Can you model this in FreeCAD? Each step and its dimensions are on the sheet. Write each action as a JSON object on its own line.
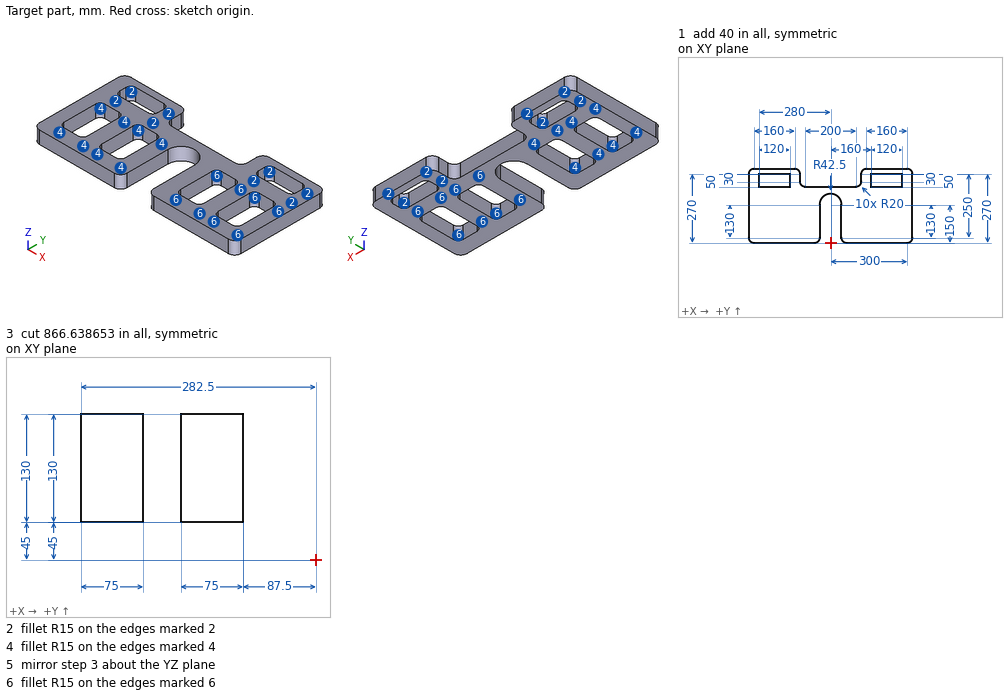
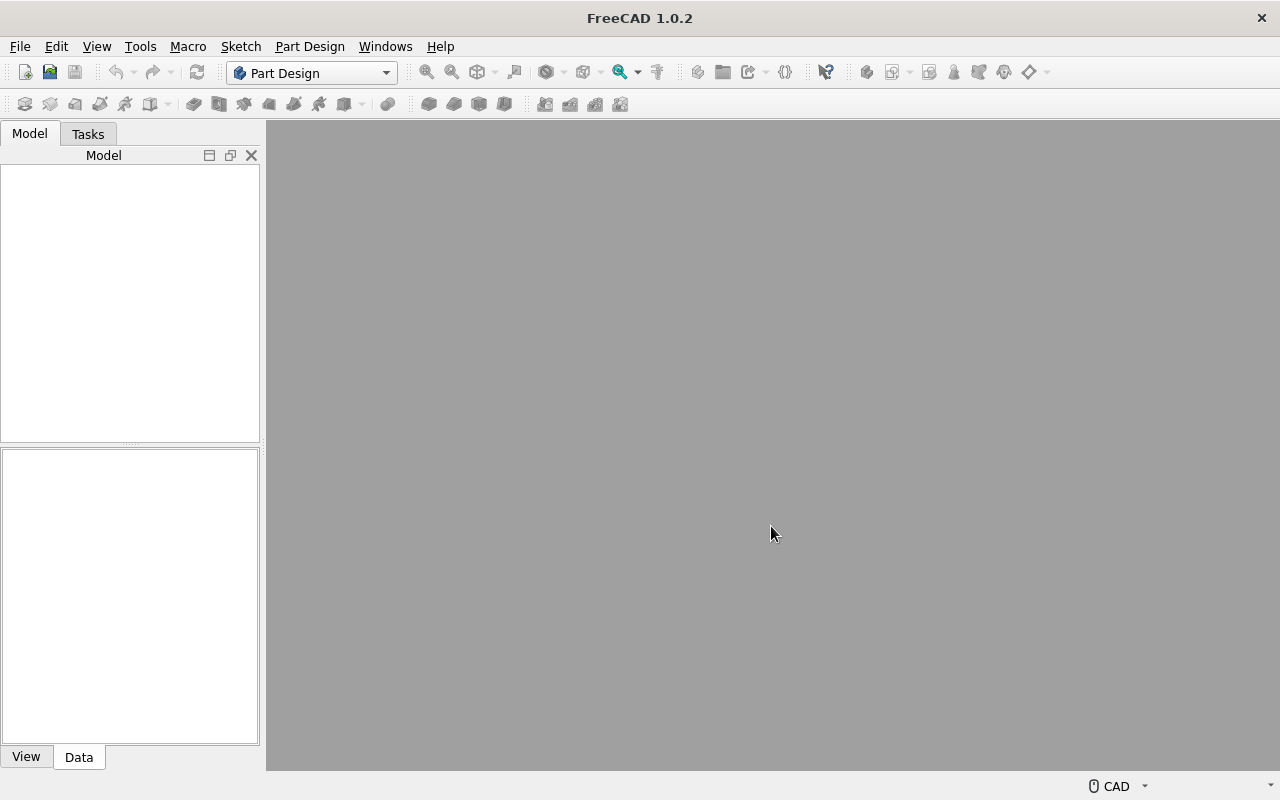
{"action": "key", "text": "ctrl+n"}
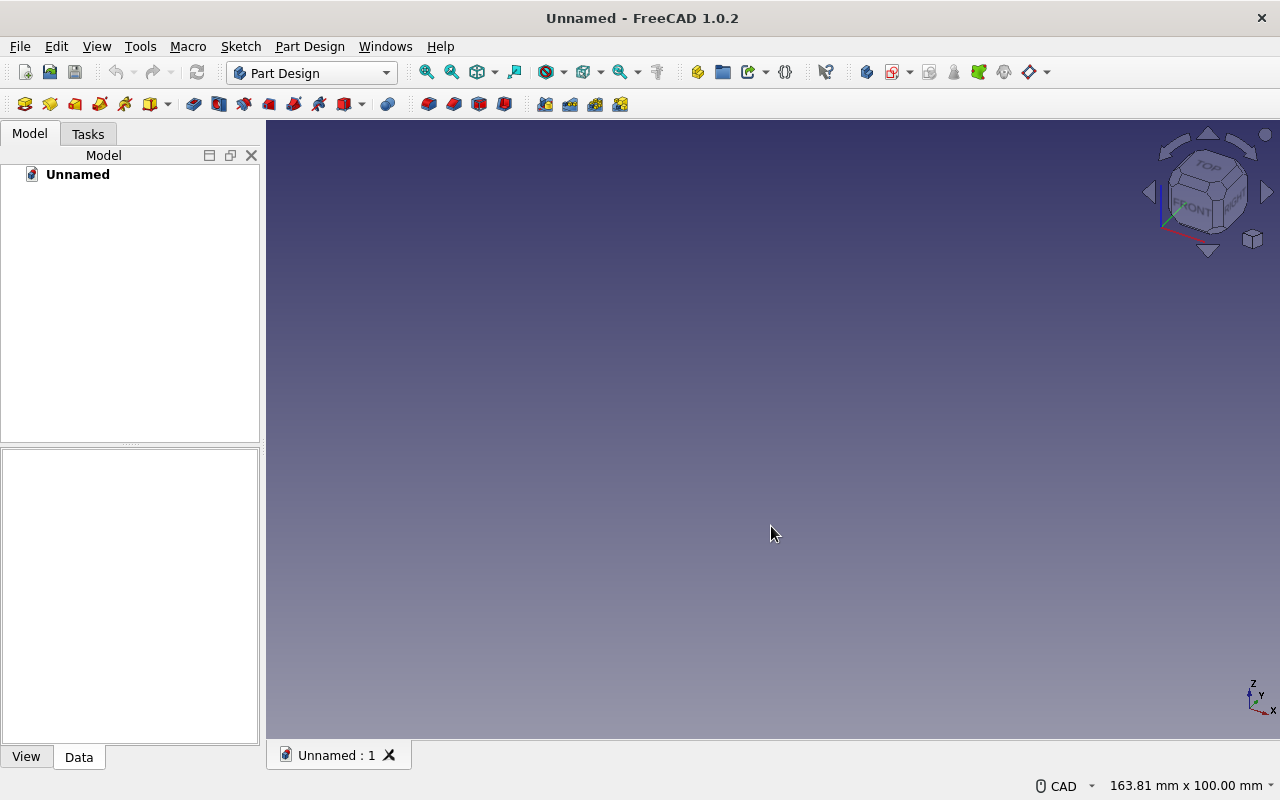
{"action": "left_click", "coordinate": [892, 72]}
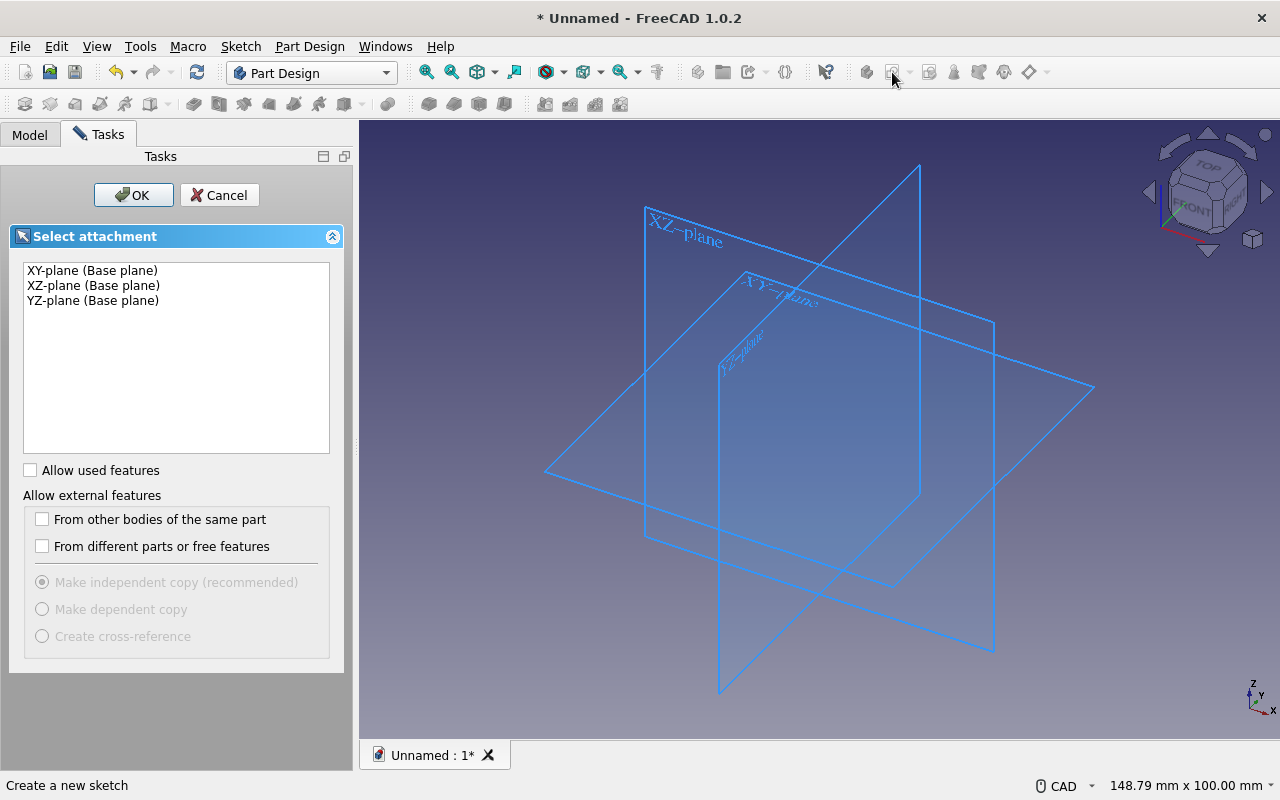
{"action": "left_click", "coordinate": [84, 270]}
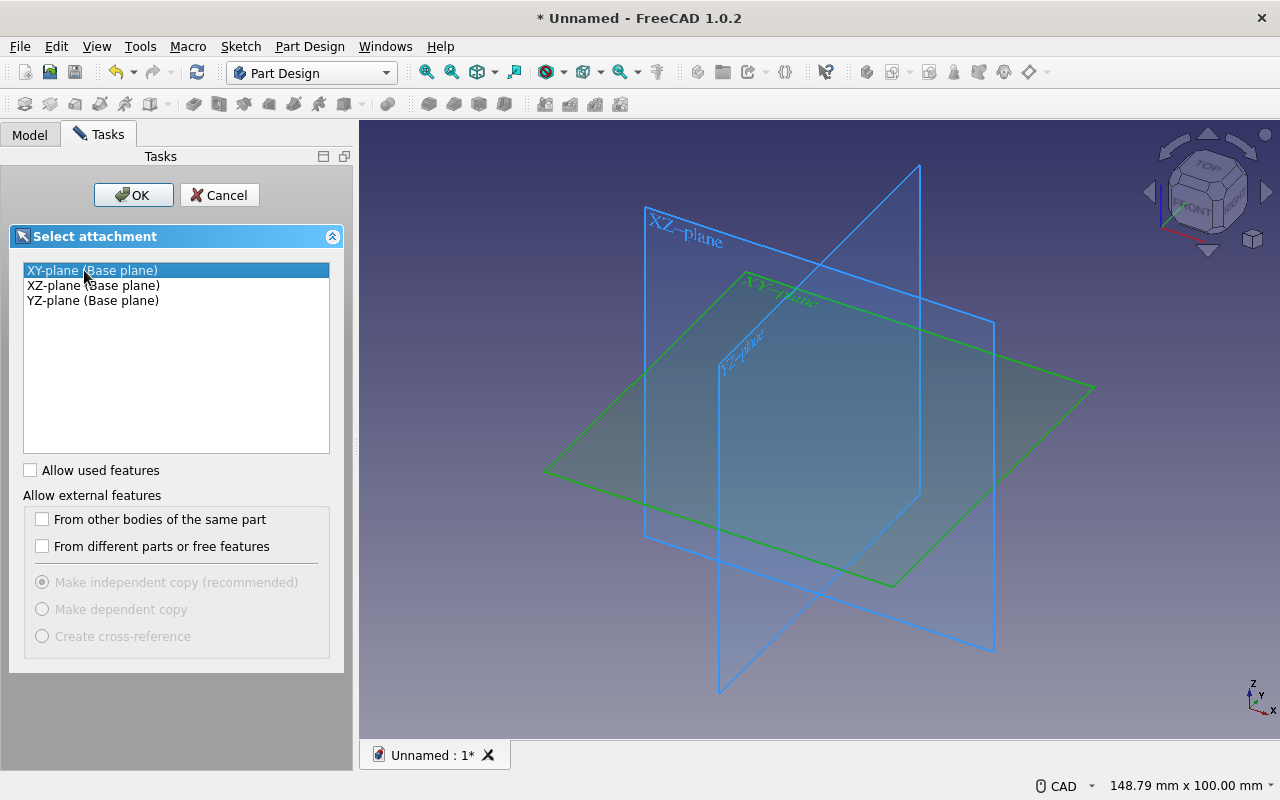
{"action": "left_click", "coordinate": [134, 195]}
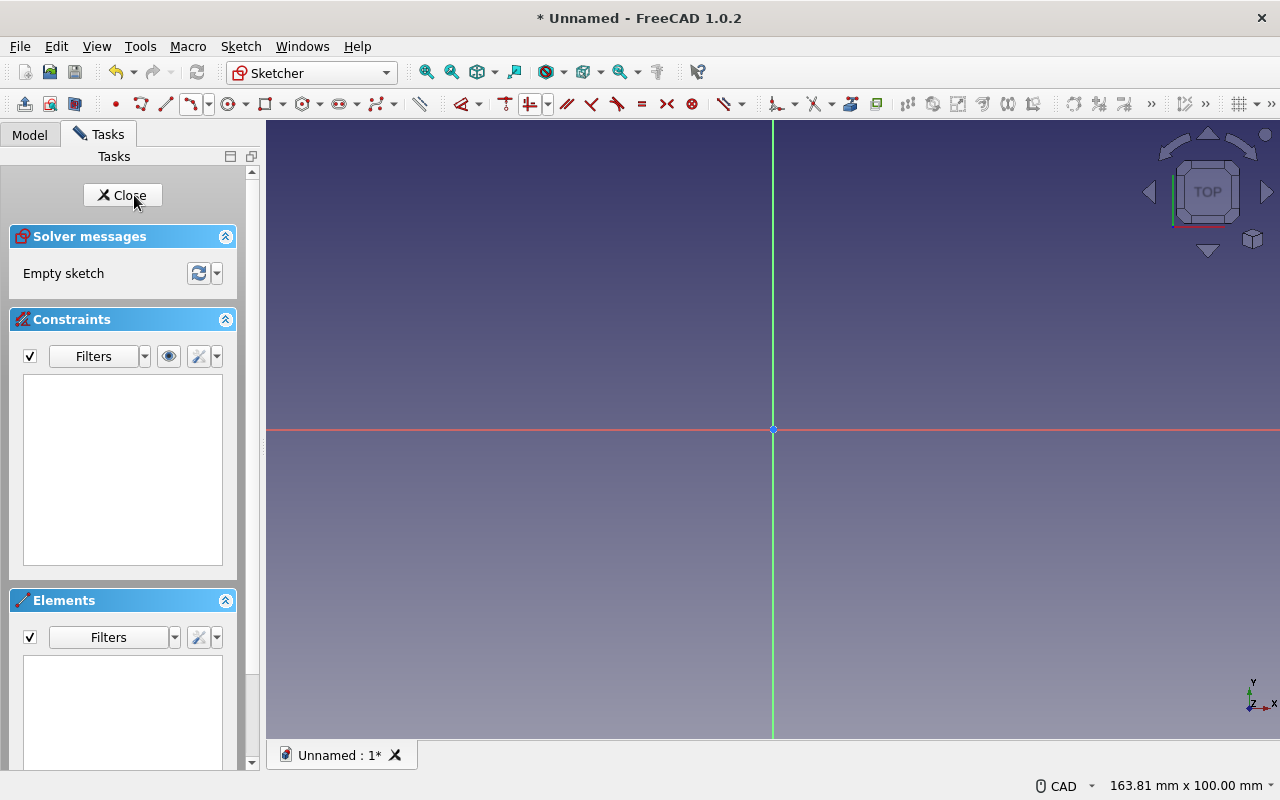
{"action": "scroll", "coordinate": [694, 570], "scroll_direction": "down", "scroll_amount": 10}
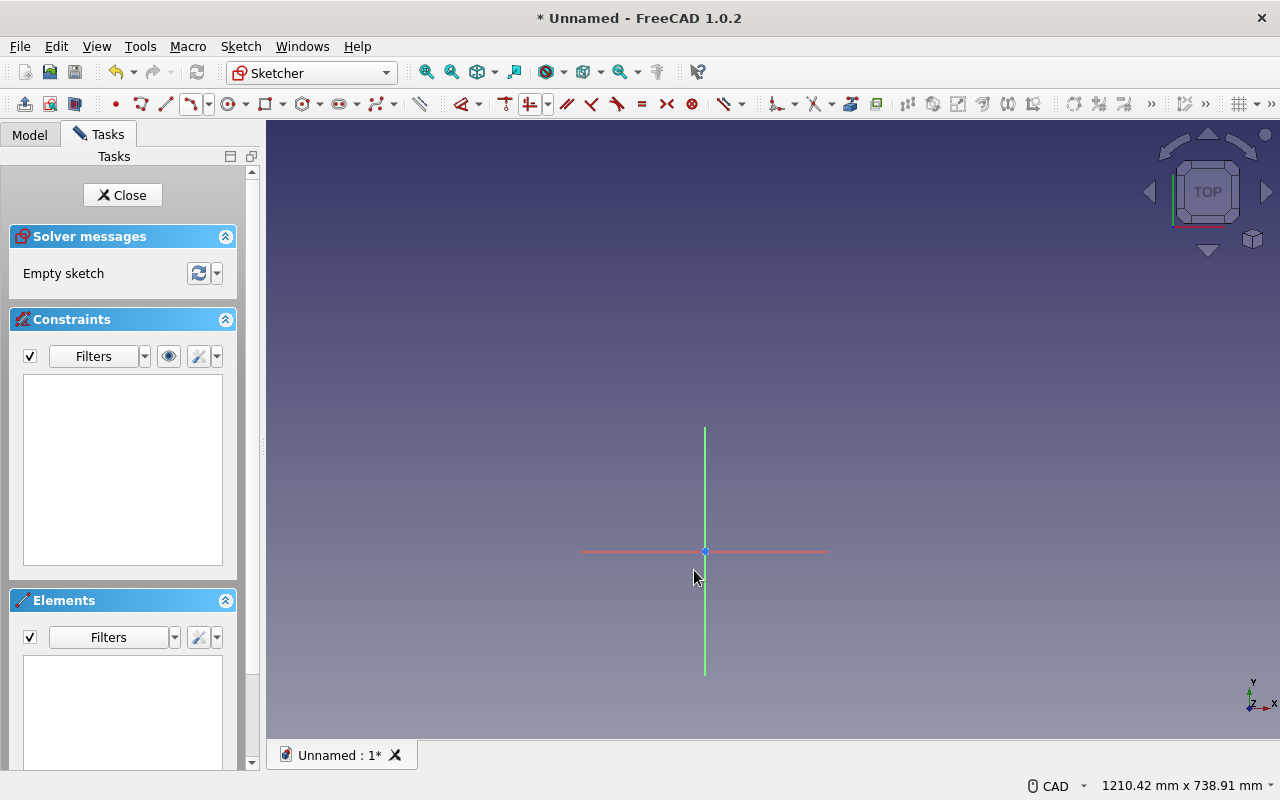
{"action": "key", "text": "g l"}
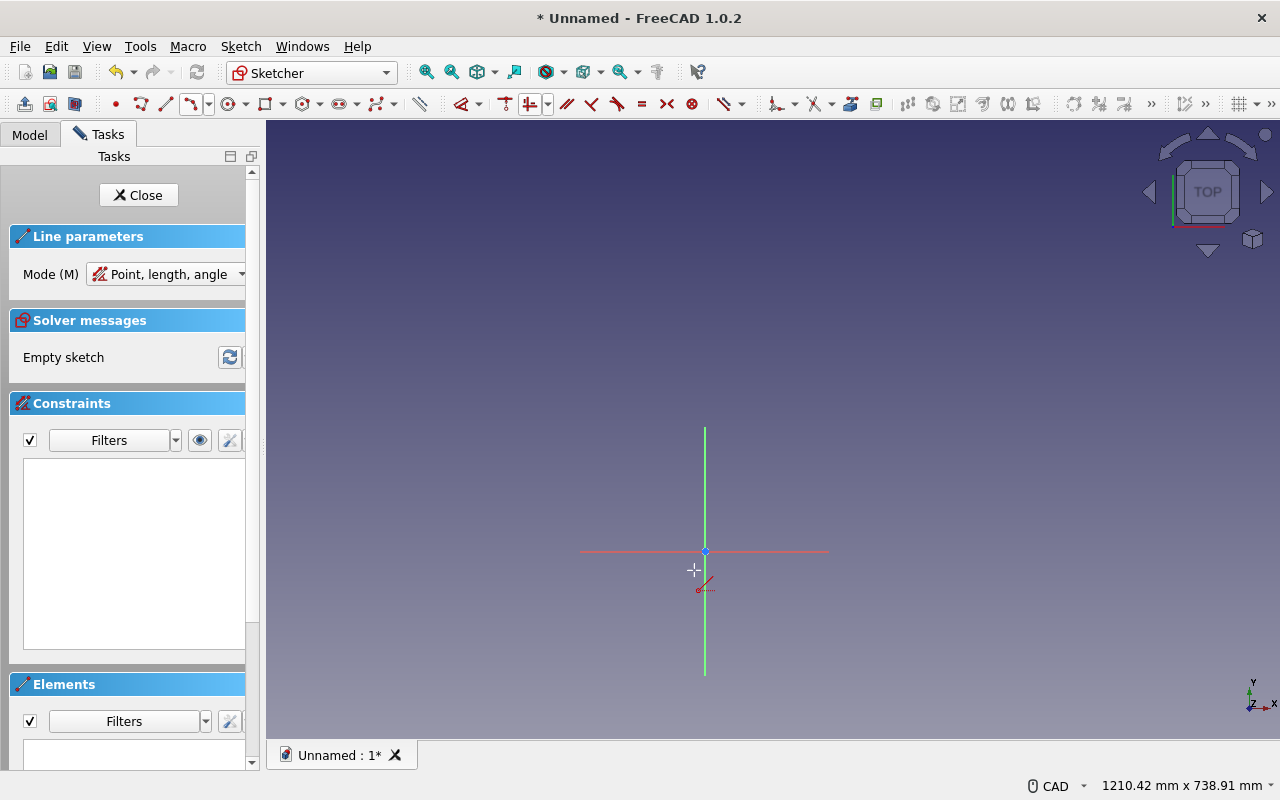
{"action": "left_click", "coordinate": [741, 426]}
{"action": "left_click", "coordinate": [741, 535]}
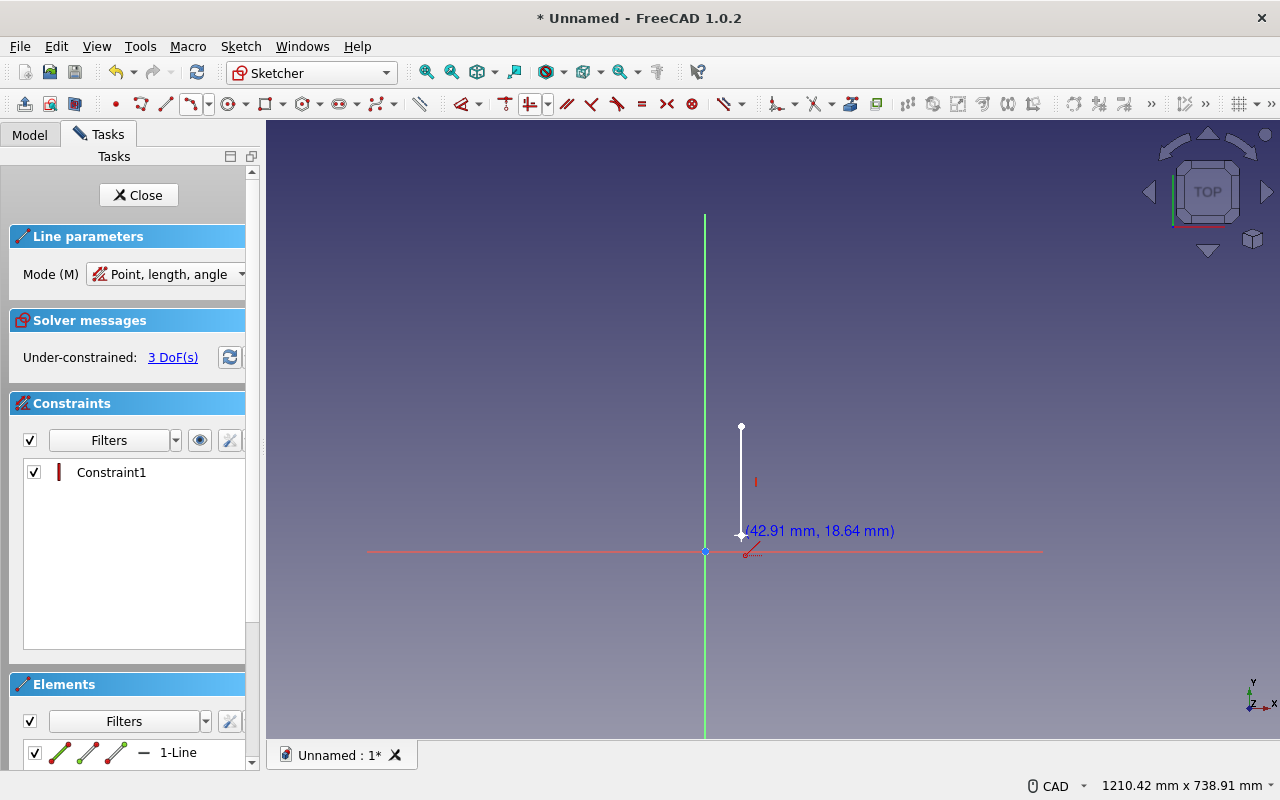
{"action": "left_click", "coordinate": [757, 552]}
{"action": "left_click", "coordinate": [956, 543]}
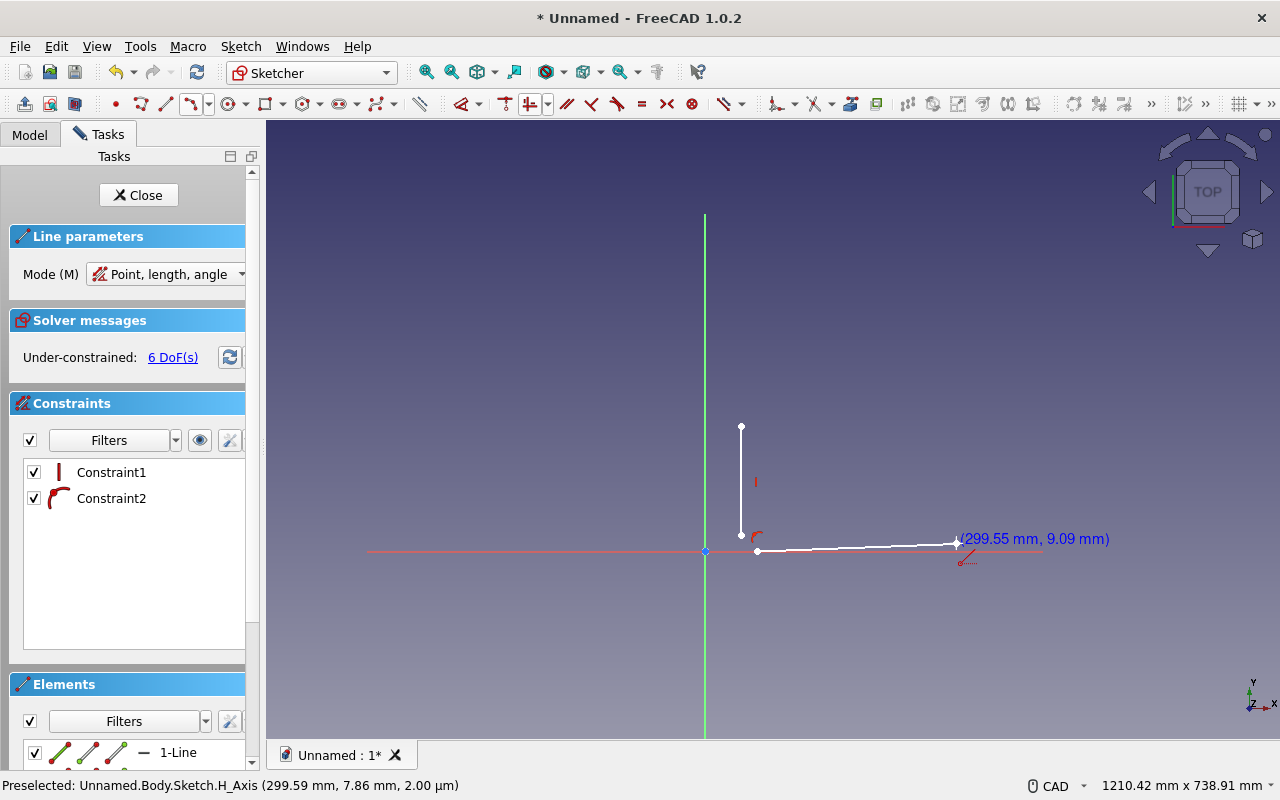
{"action": "left_click", "coordinate": [973, 535]}
{"action": "left_click", "coordinate": [973, 325]}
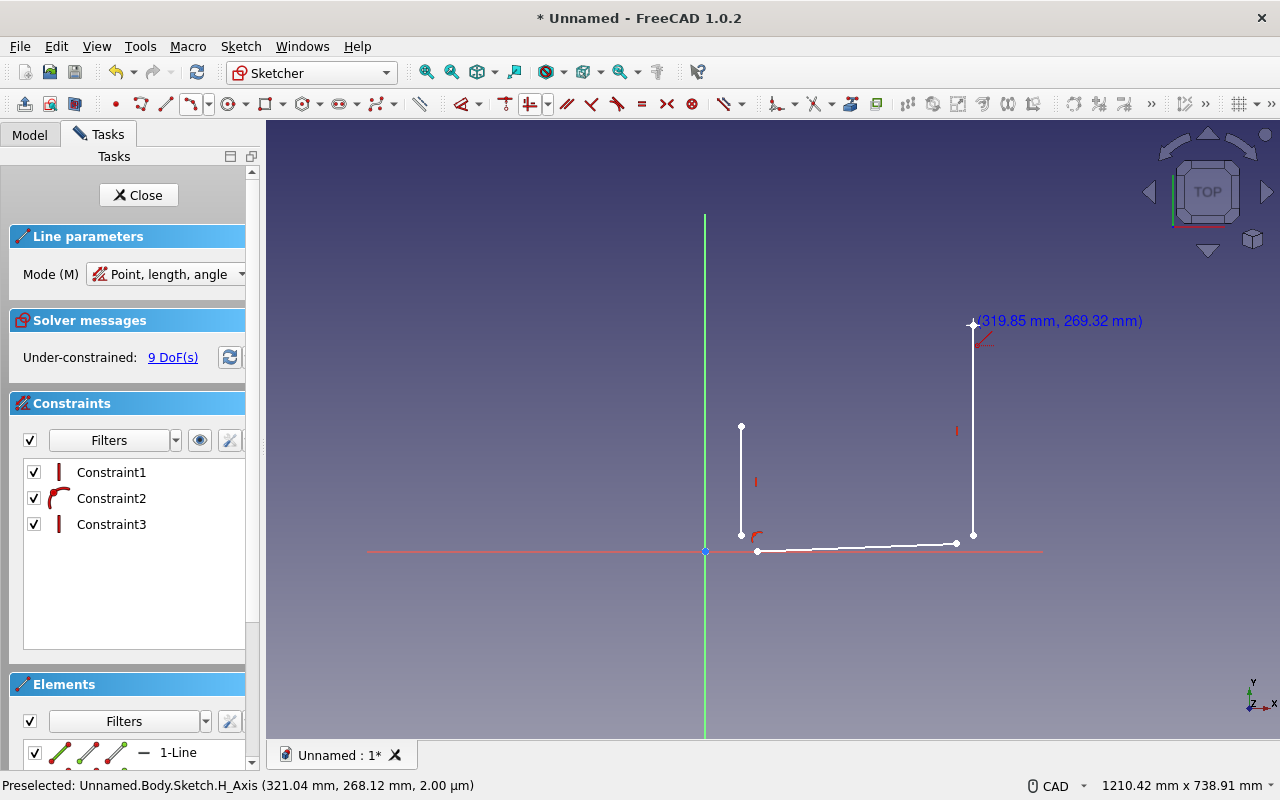
{"action": "left_click", "coordinate": [956, 309]}
{"action": "left_click", "coordinate": [822, 309]}